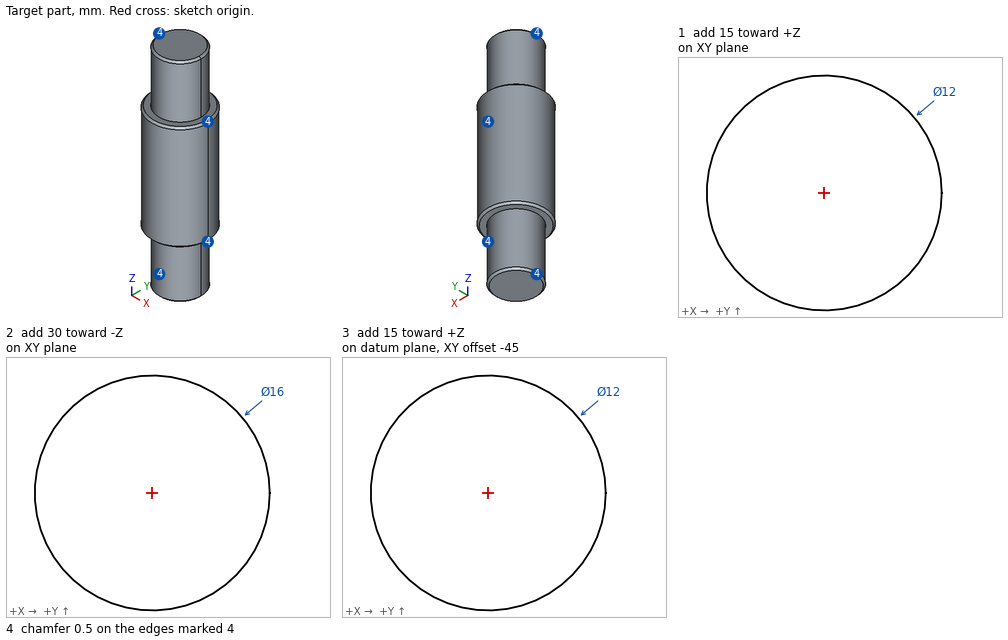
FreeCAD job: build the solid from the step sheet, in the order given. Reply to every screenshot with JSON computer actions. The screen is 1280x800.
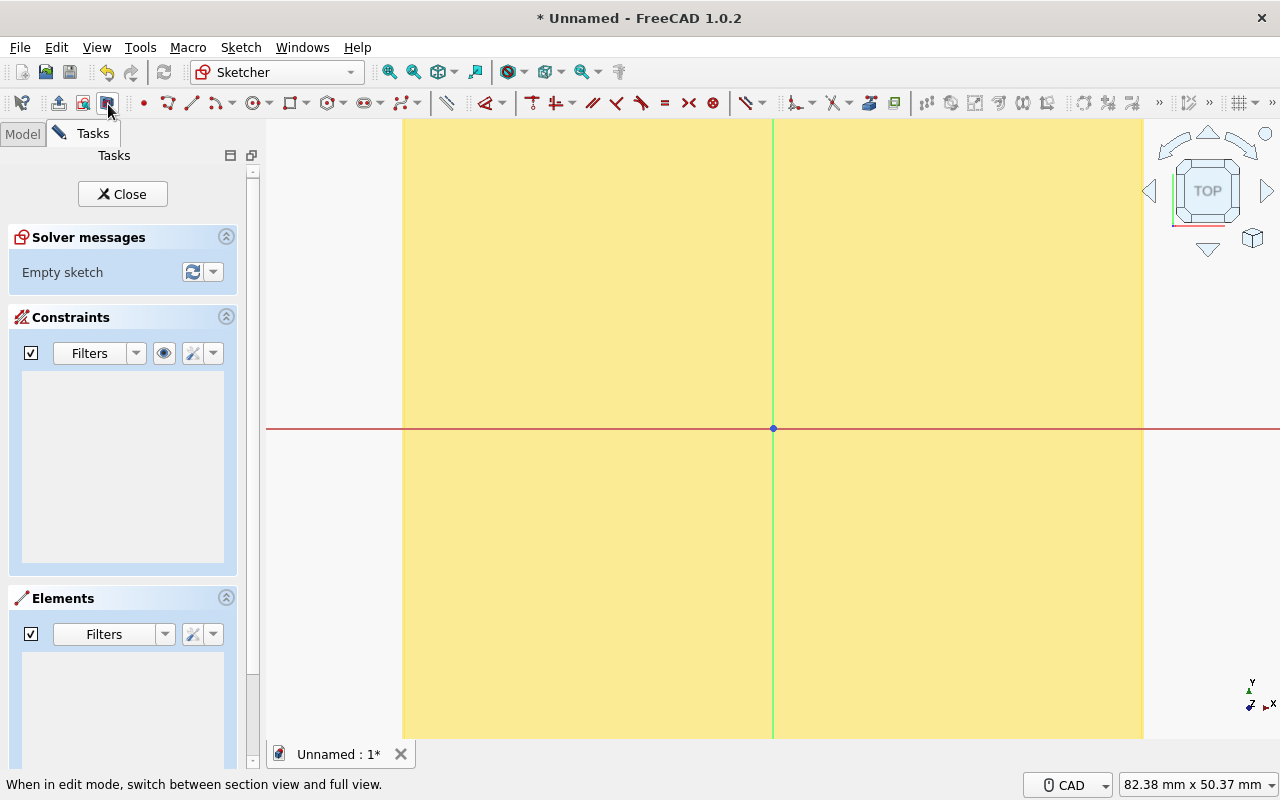
{"action": "scroll", "coordinate": [813, 429], "scroll_direction": "up", "scroll_amount": 5}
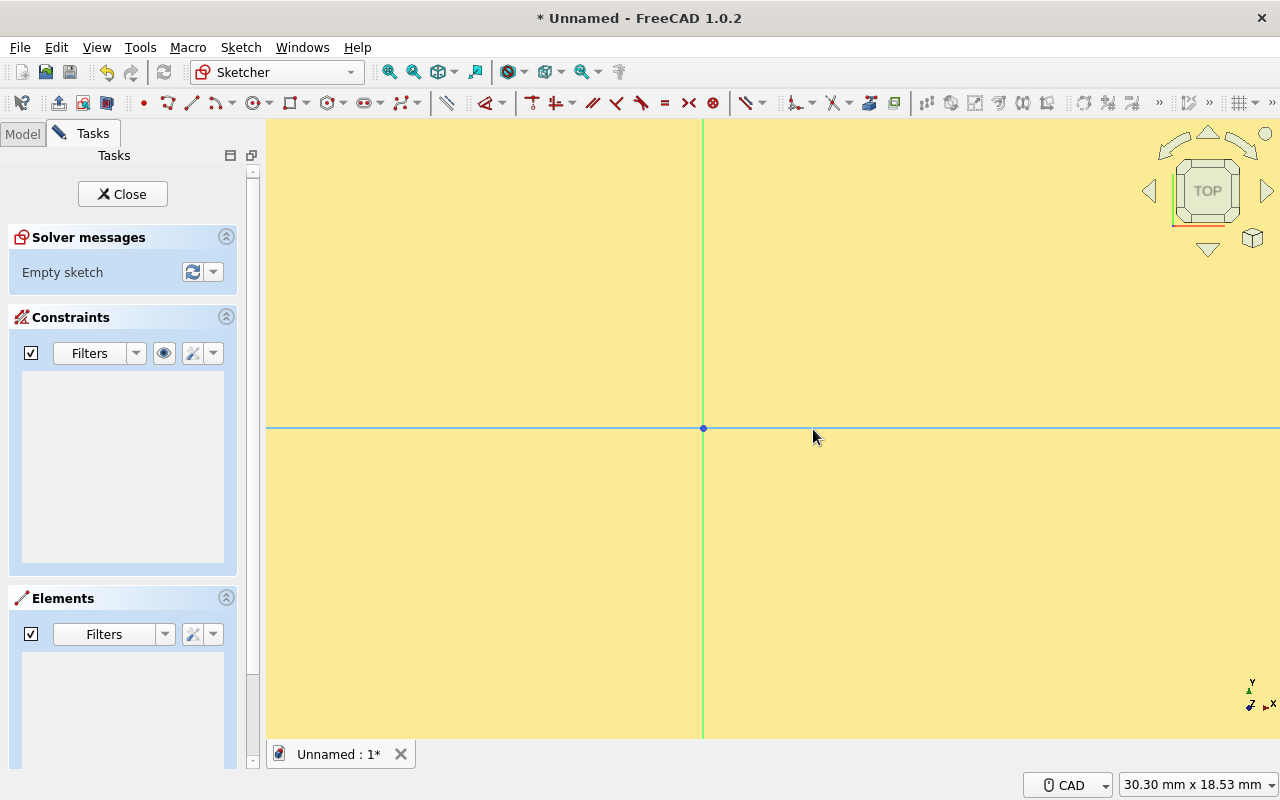
{"action": "left_click", "coordinate": [254, 104]}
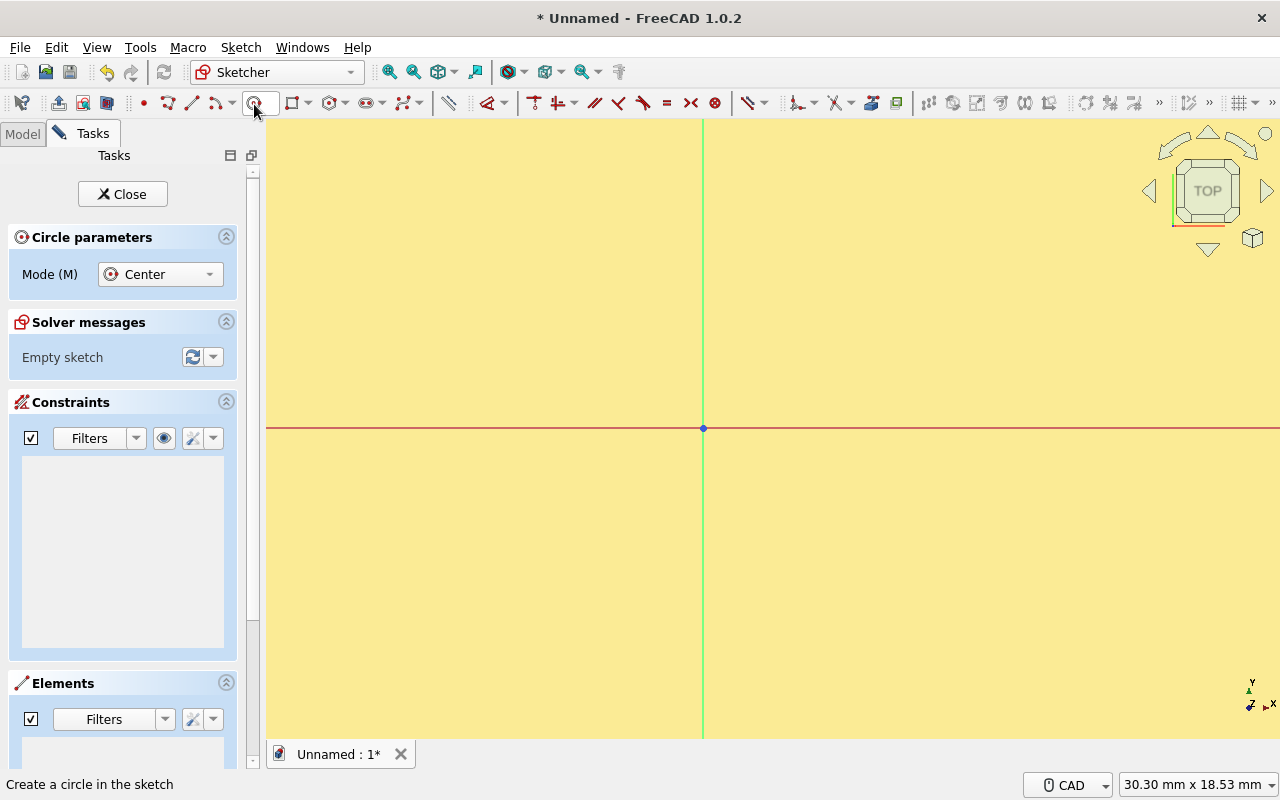
{"action": "left_click", "coordinate": [703, 428]}
{"action": "left_click", "coordinate": [845, 286]}
{"action": "key", "text": "Escape"}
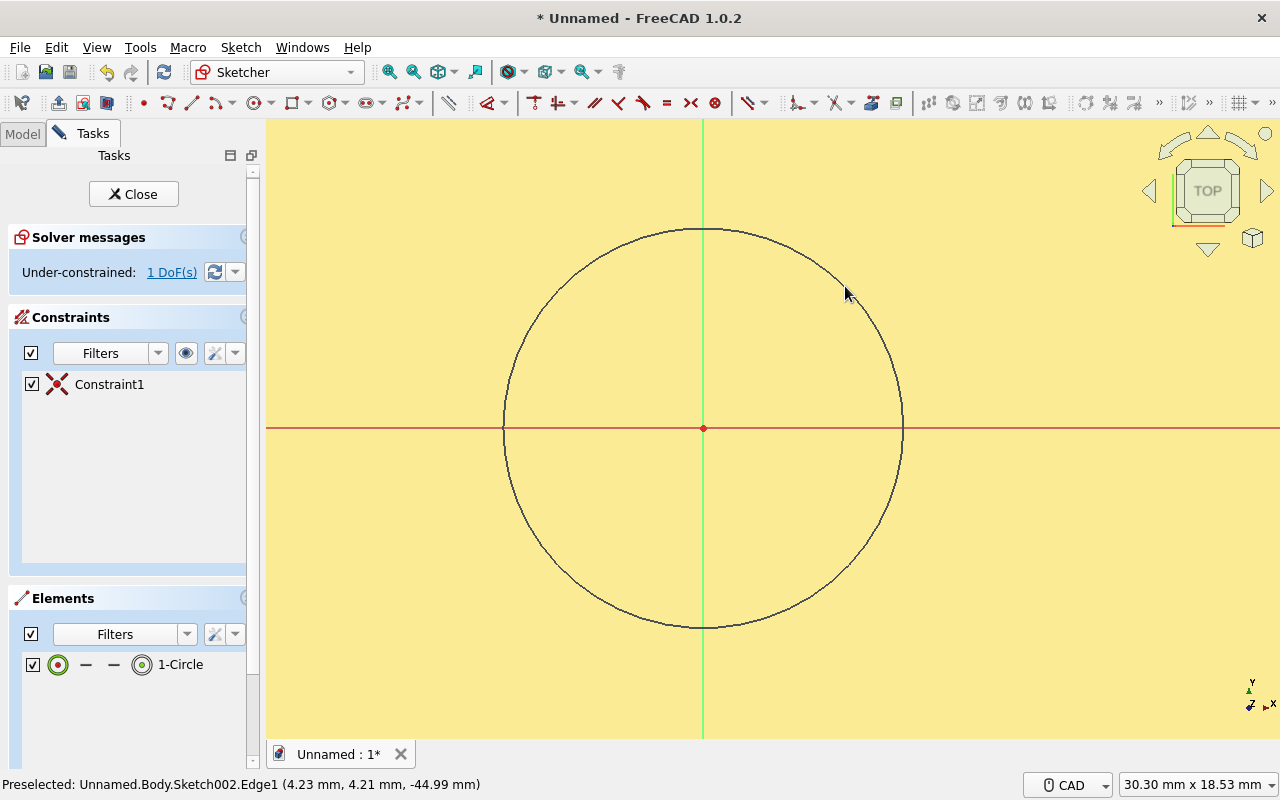
{"action": "left_click", "coordinate": [488, 104]}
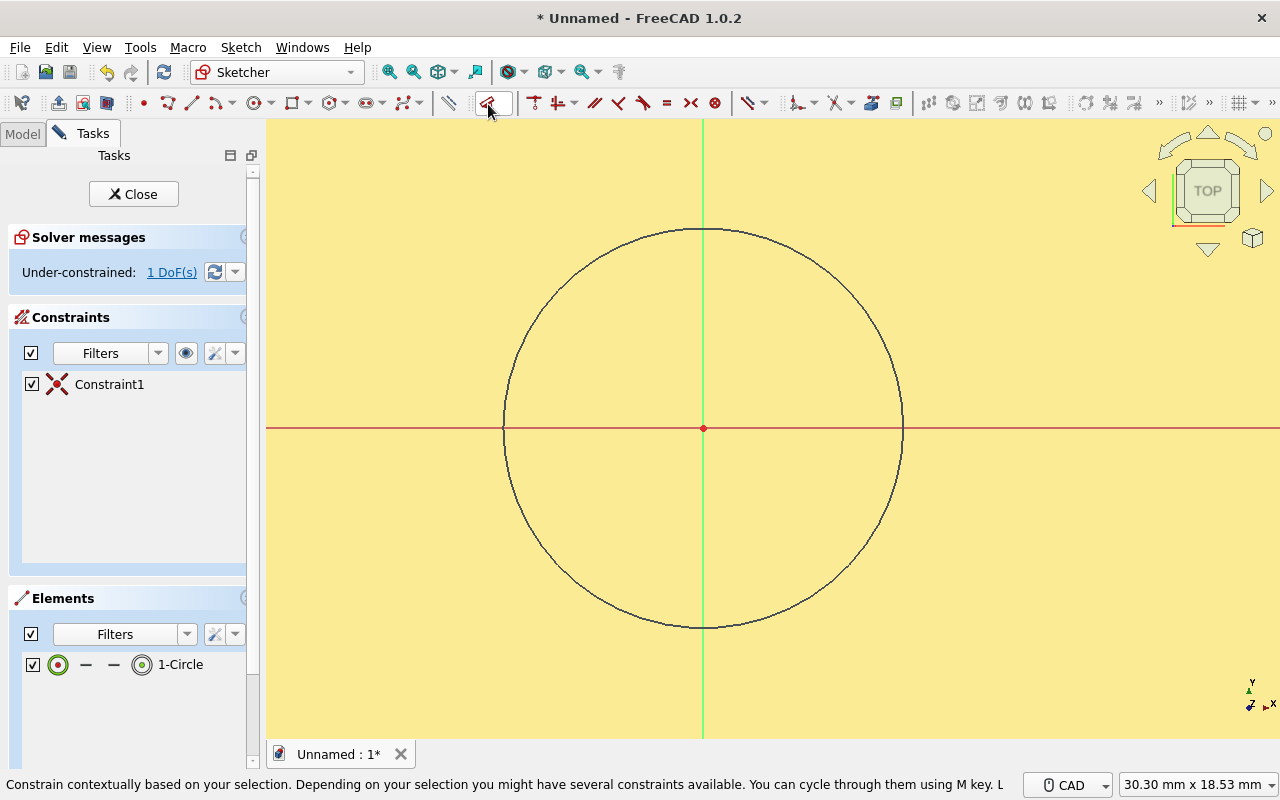
{"action": "left_click", "coordinate": [844, 286]}
{"action": "left_click", "coordinate": [867, 263]}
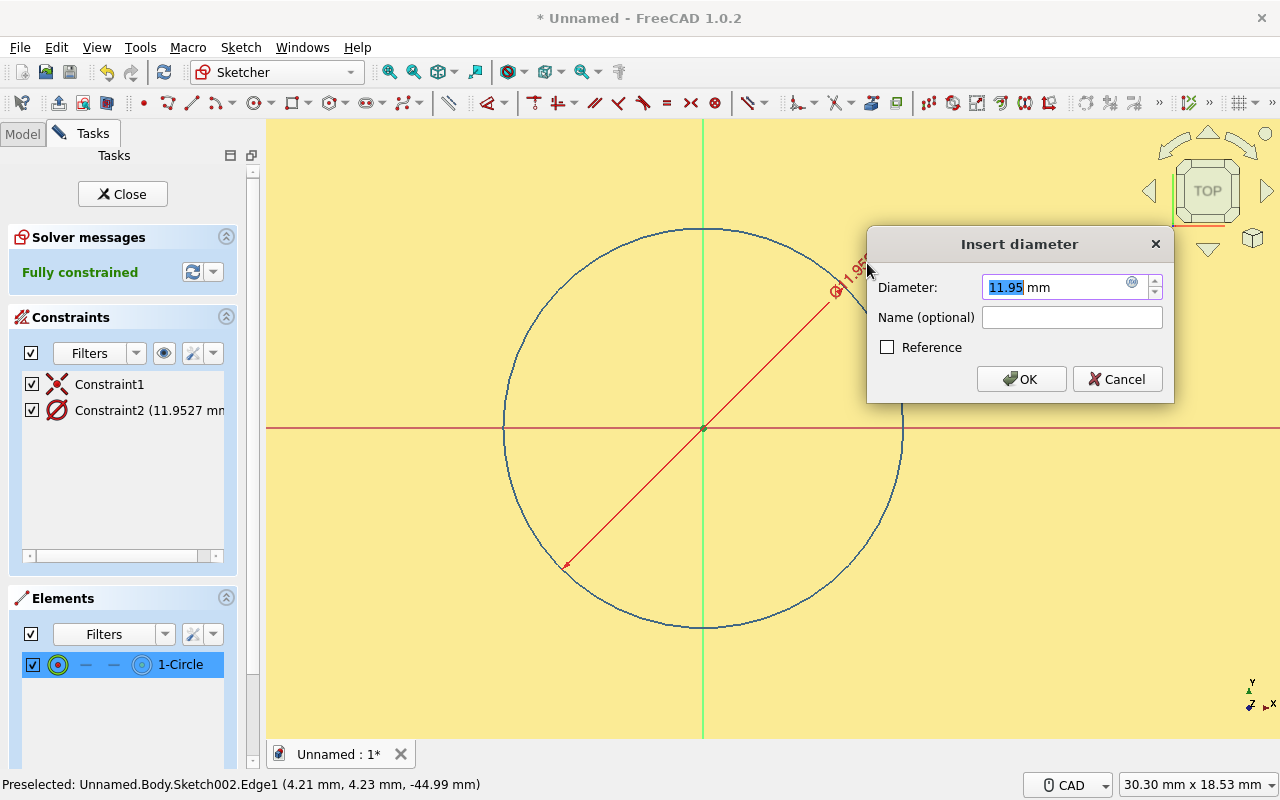
{"action": "type", "text": "12"}
{"action": "key", "text": "Return"}
{"action": "key", "text": "Escape"}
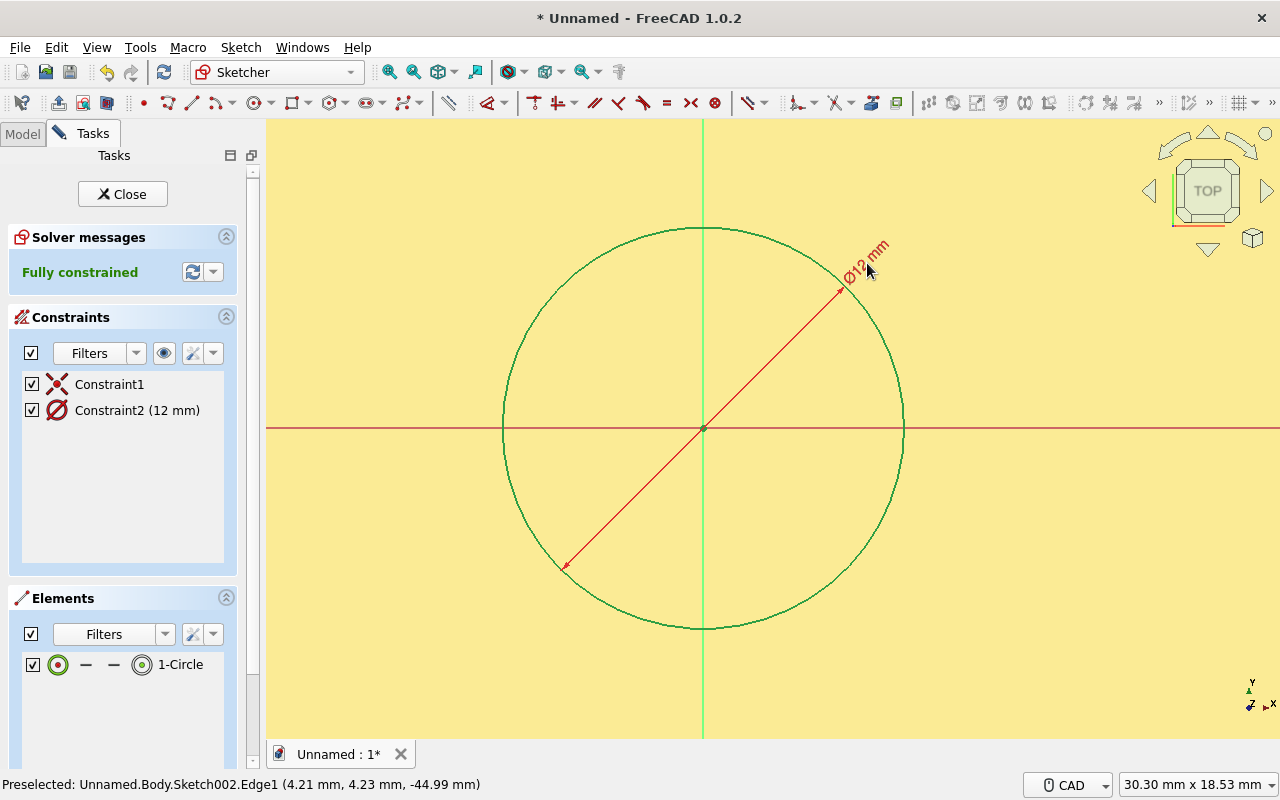
{"action": "left_click", "coordinate": [123, 194]}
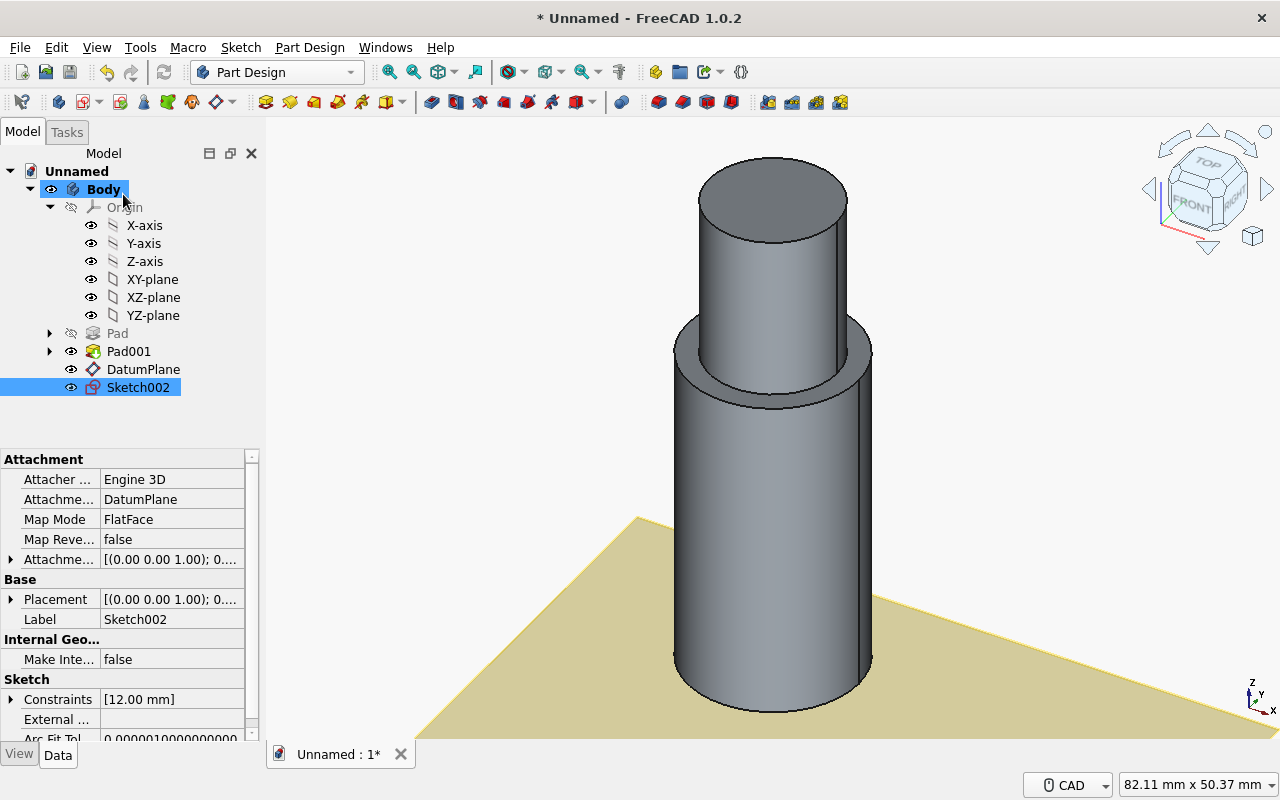
{"action": "left_click", "coordinate": [266, 102]}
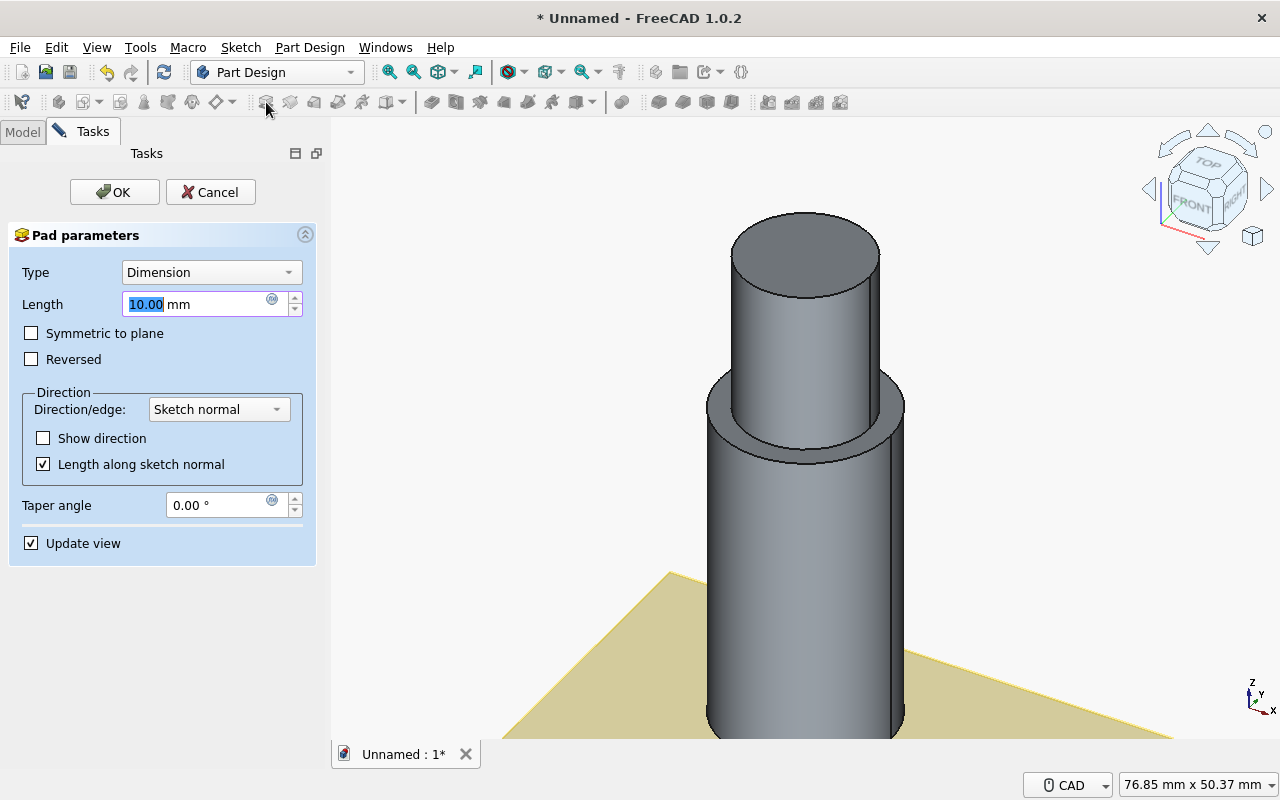
{"action": "type", "text": "15"}
{"action": "key", "text": "Tab"}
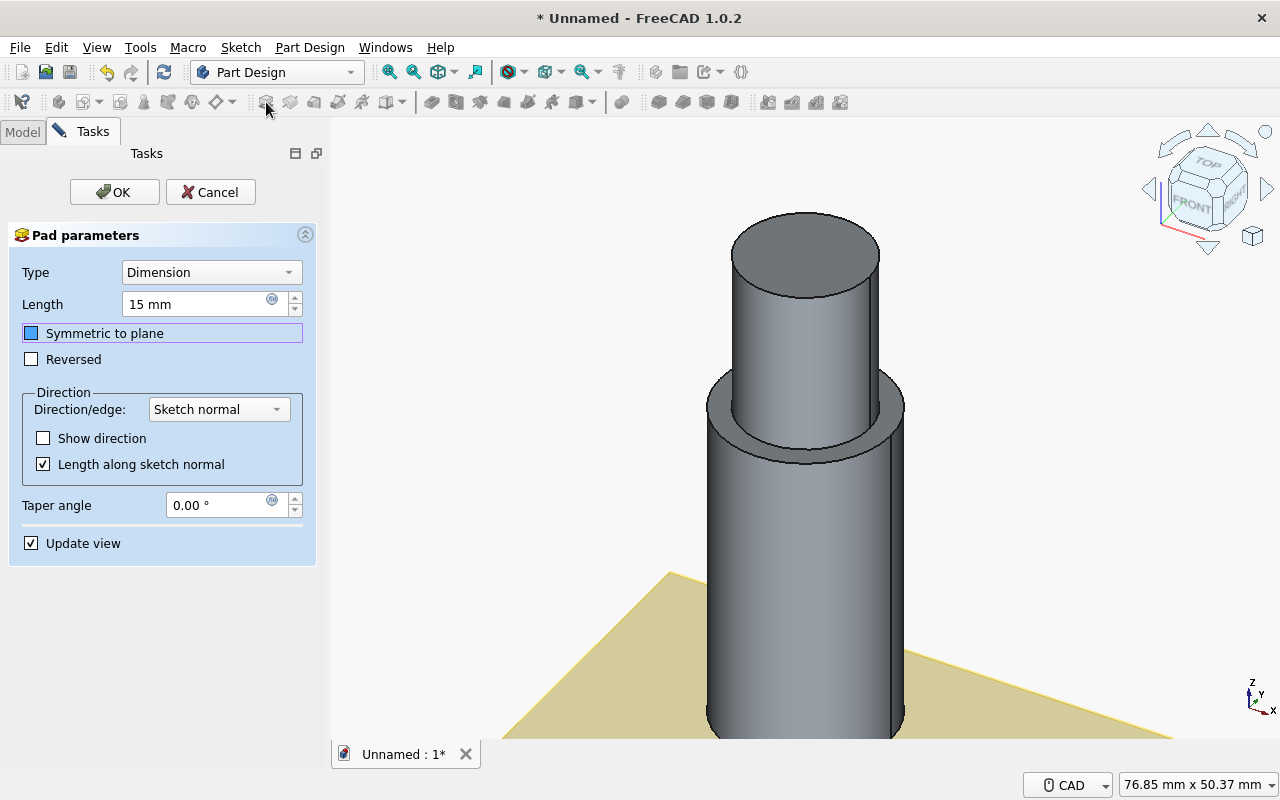
{"action": "left_click", "coordinate": [115, 192]}